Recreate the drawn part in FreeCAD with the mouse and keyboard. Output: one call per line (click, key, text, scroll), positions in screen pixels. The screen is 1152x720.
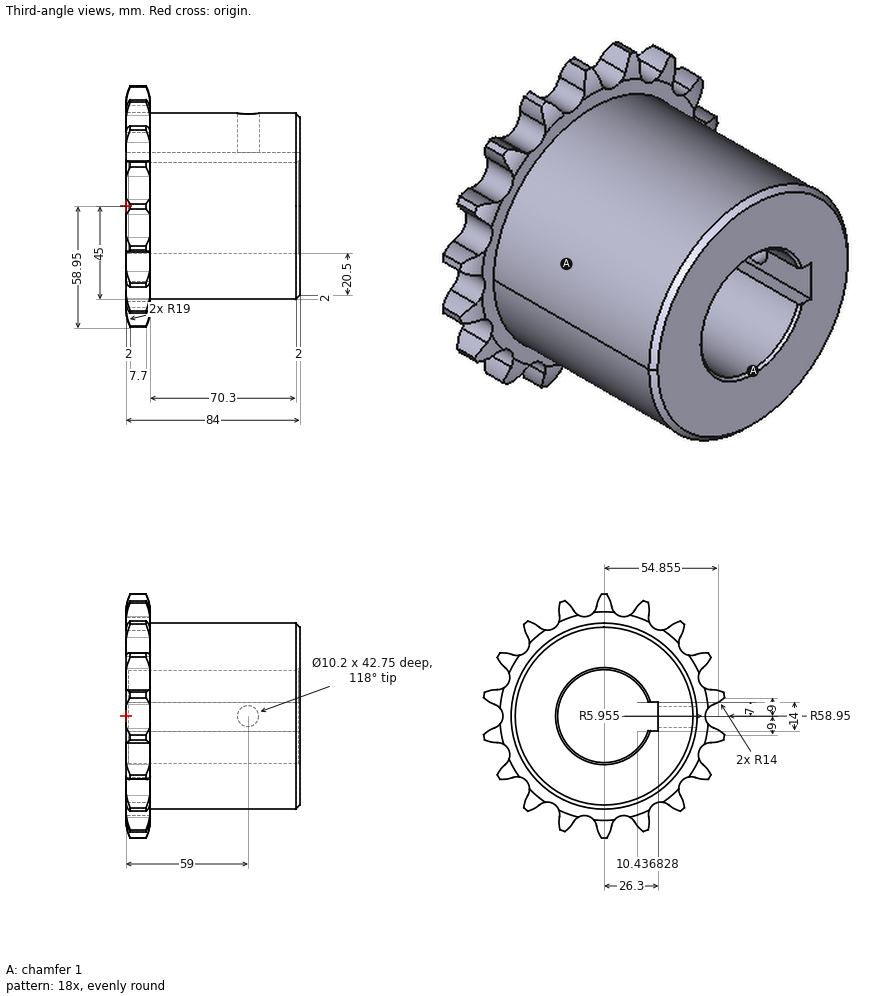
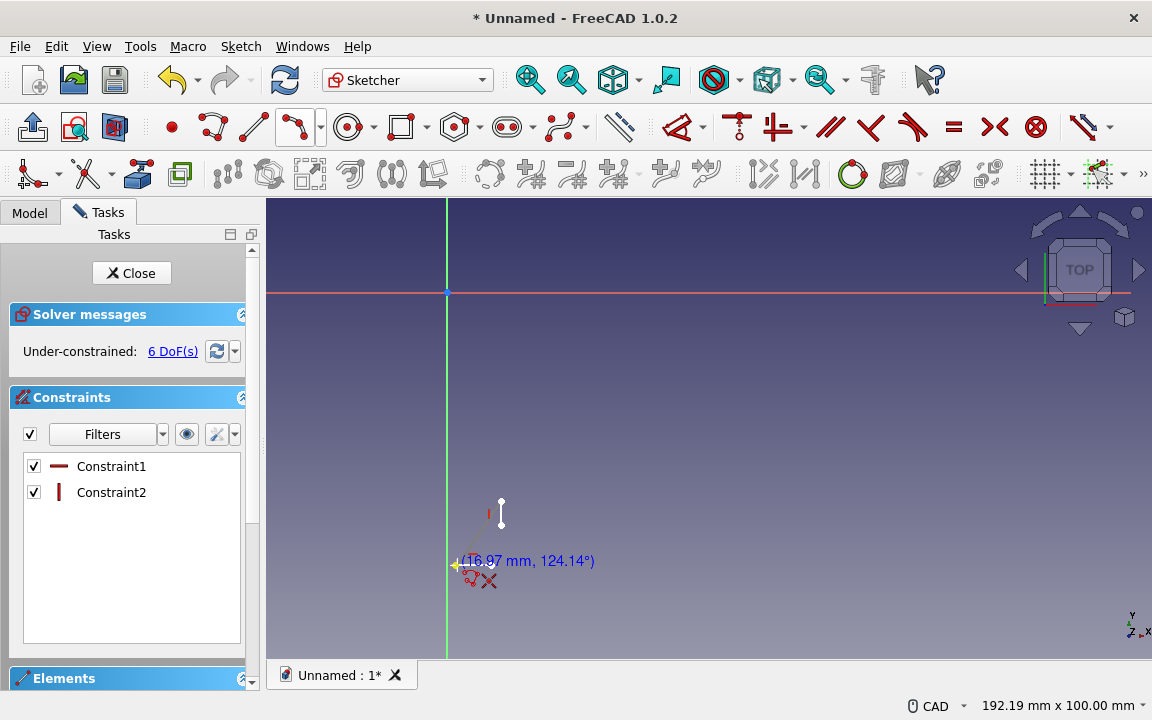
click(825, 501)
click(834, 491)
click(834, 397)
click(447, 397)
click(456, 526)
right_click(456, 526)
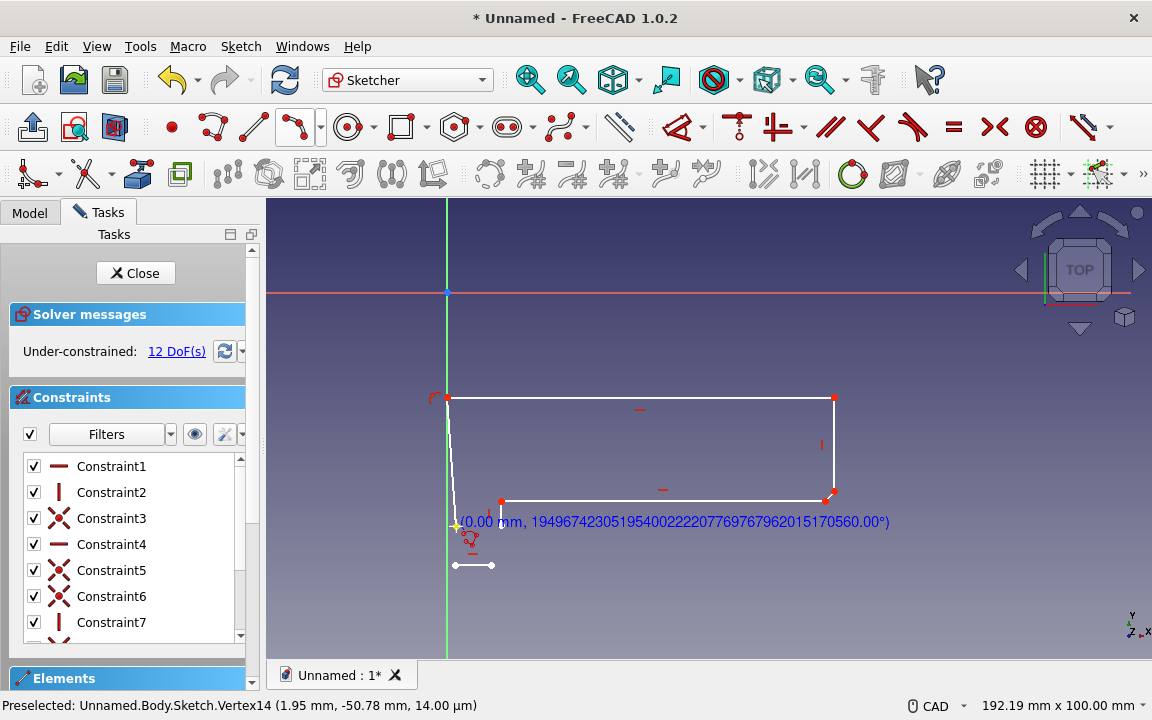
key(g)
key(3)
key(a)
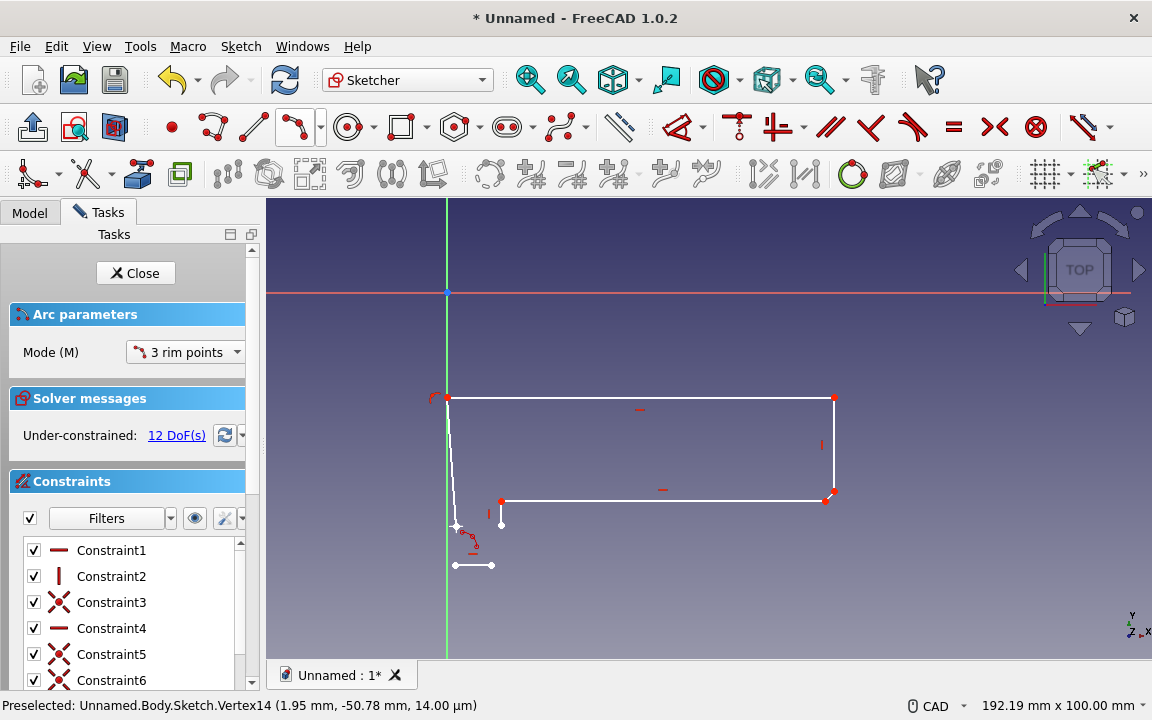
click(492, 565)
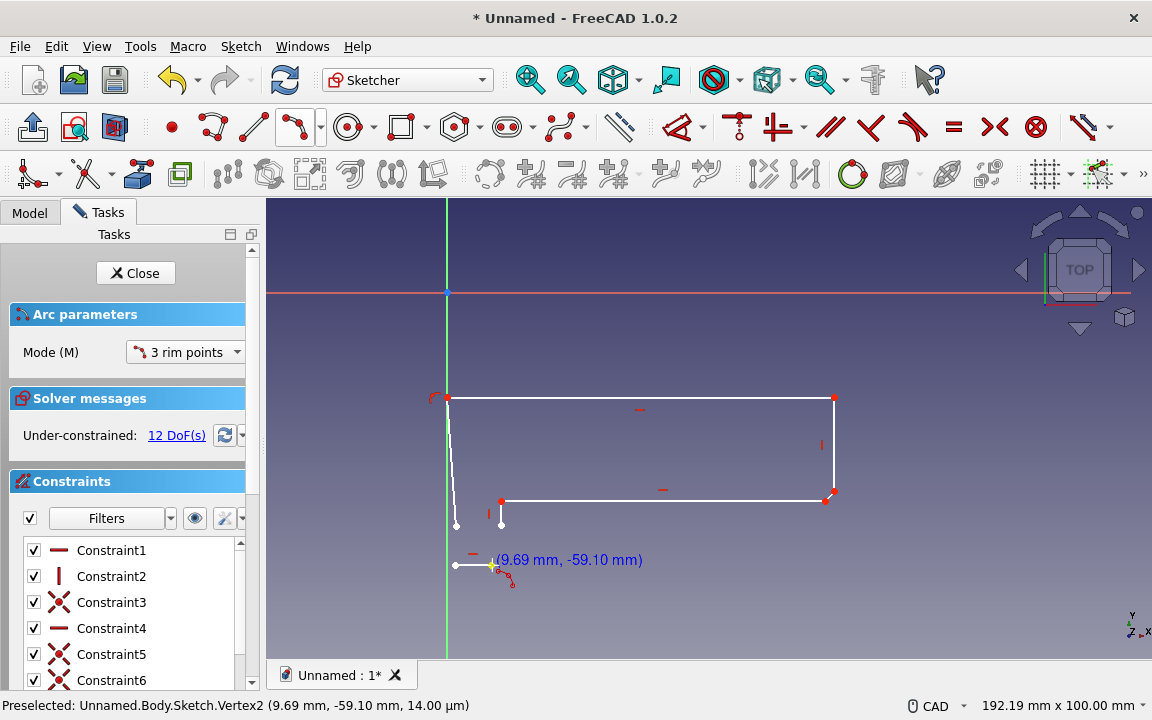
scroll(501, 526, up, 2)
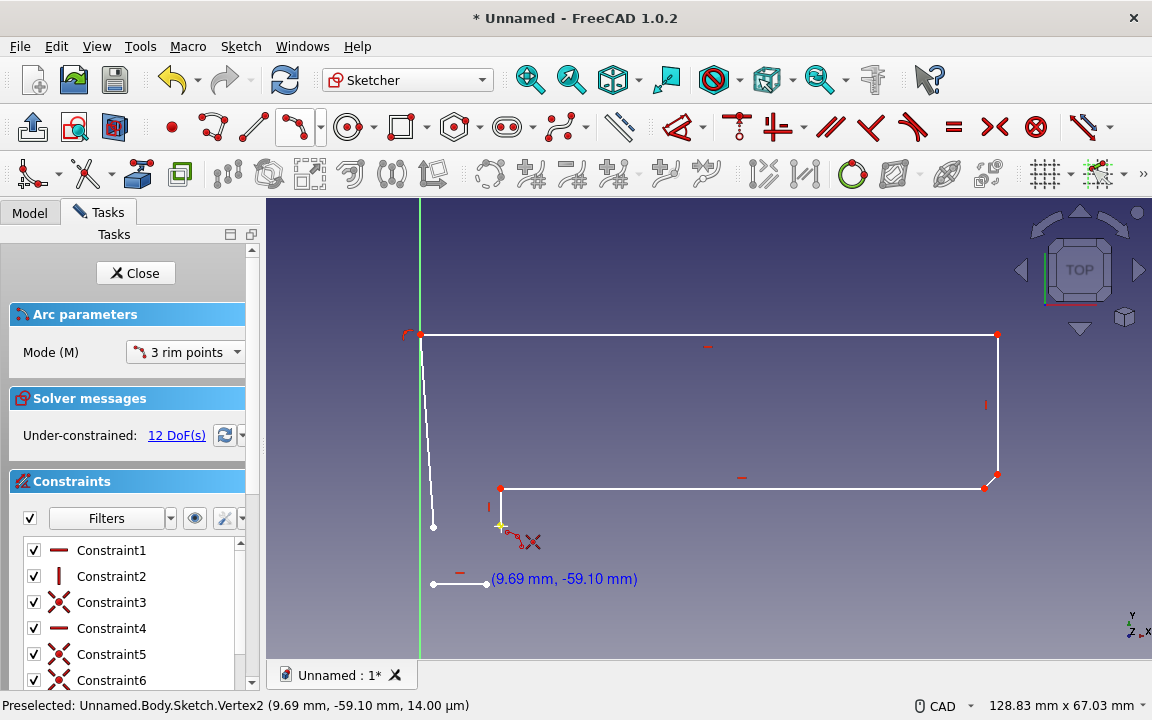
click(501, 525)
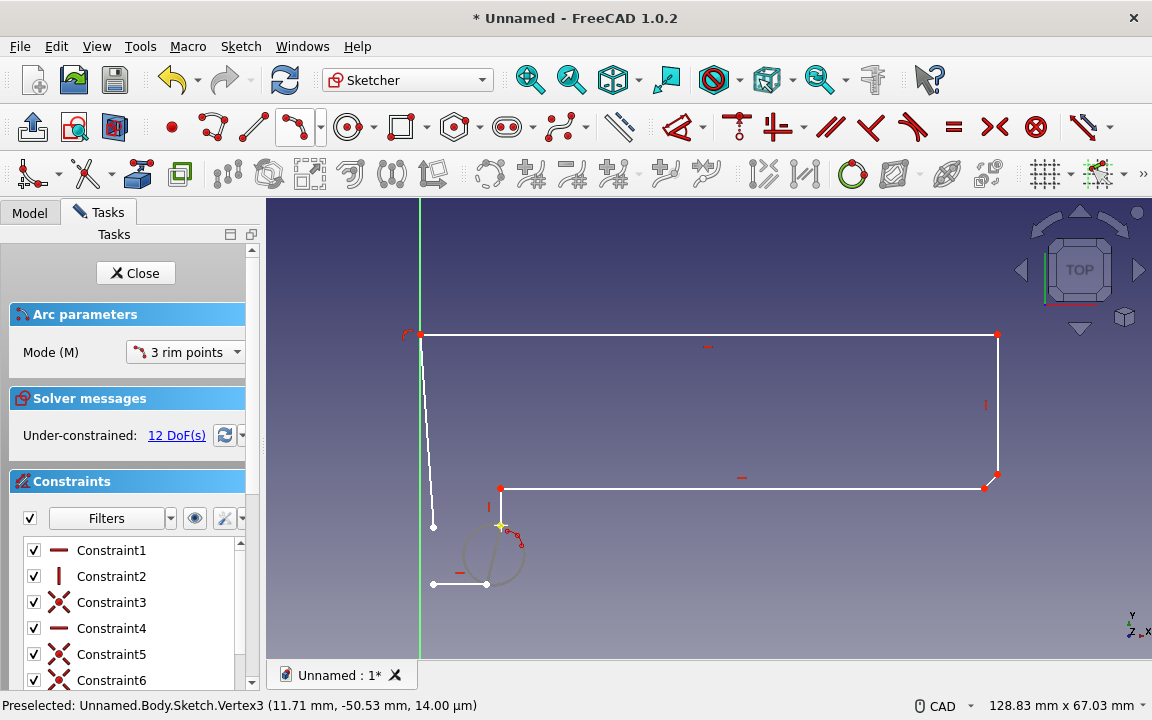
scroll(497, 555, up, 8)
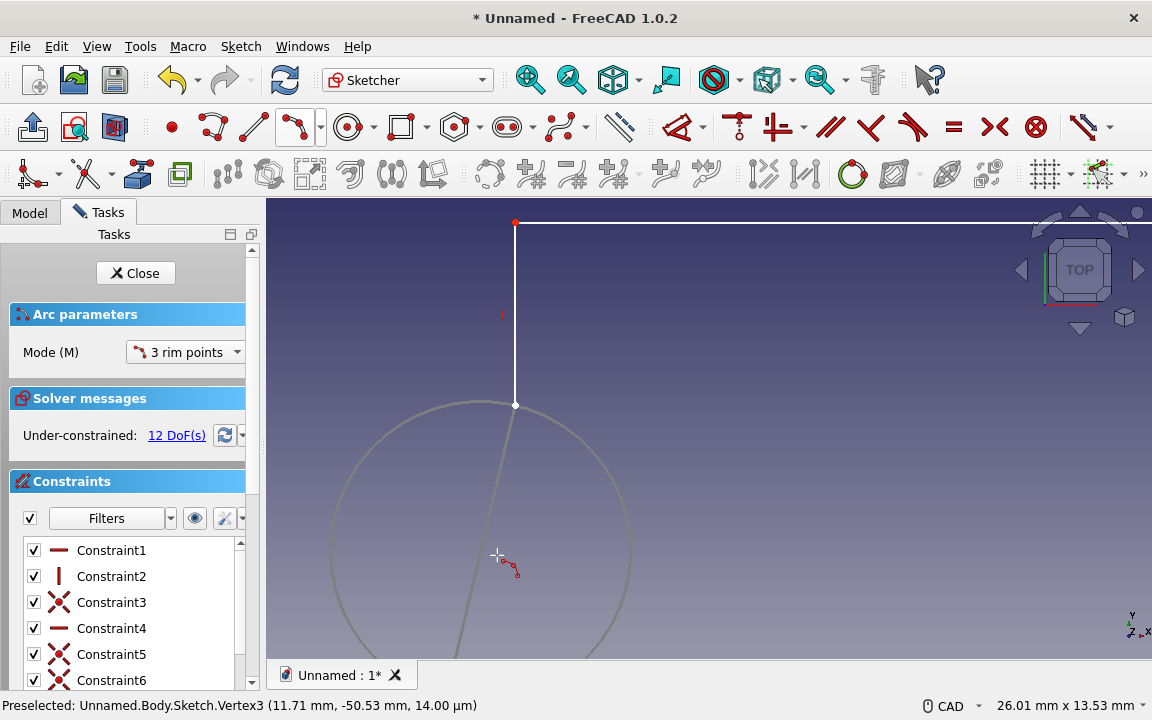
click(498, 552)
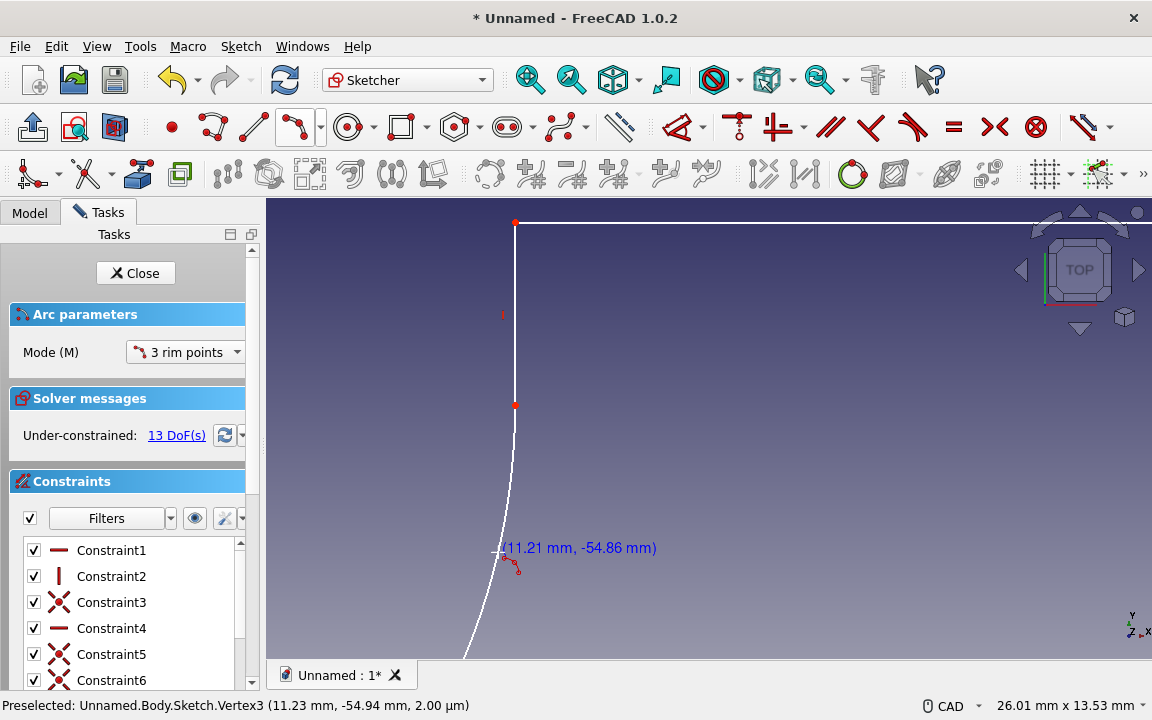
scroll(499, 544, down, 10)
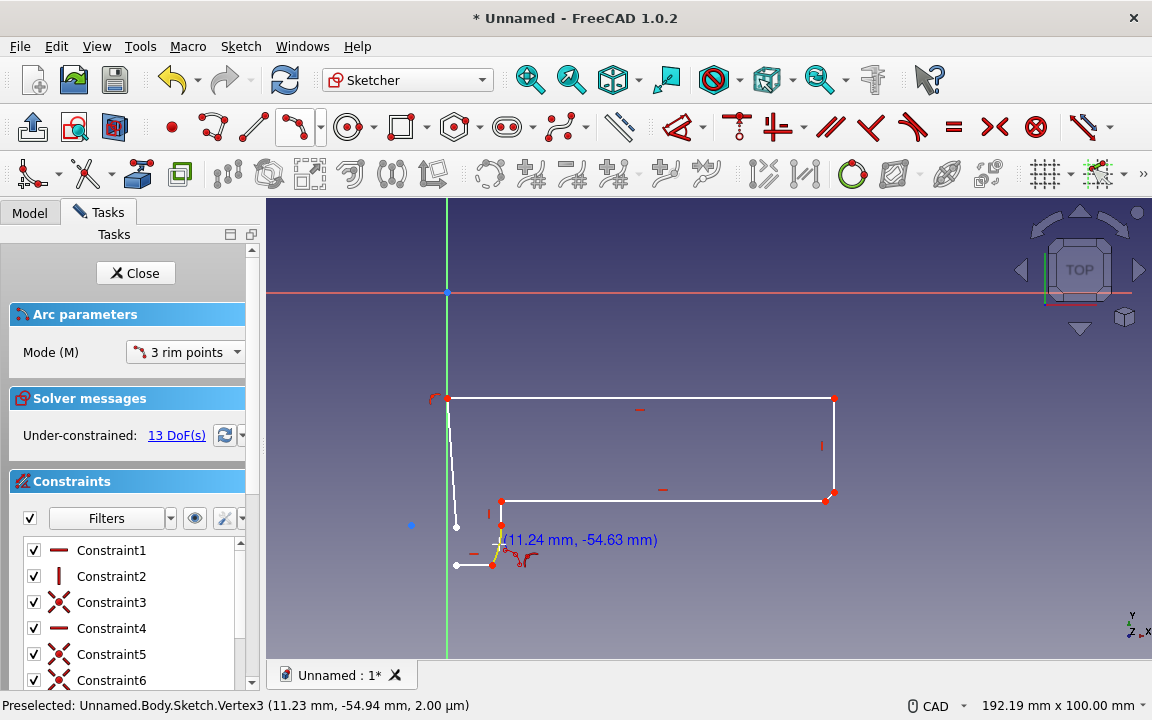
click(456, 527)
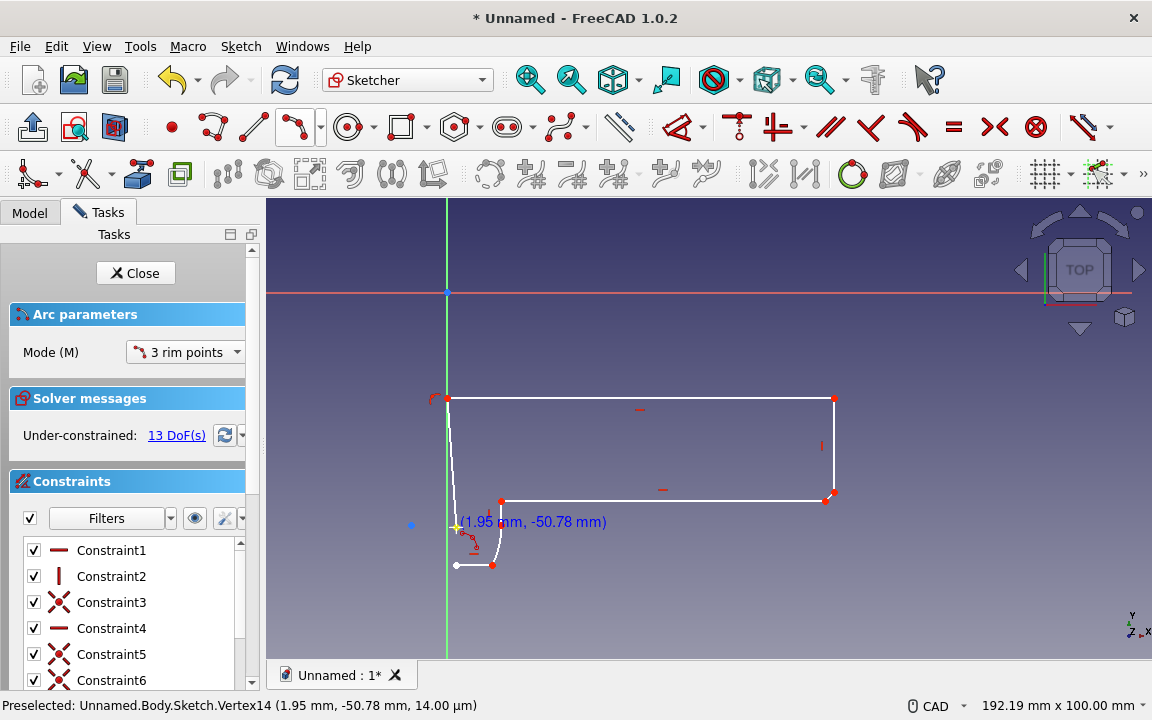
scroll(457, 565, up, 3)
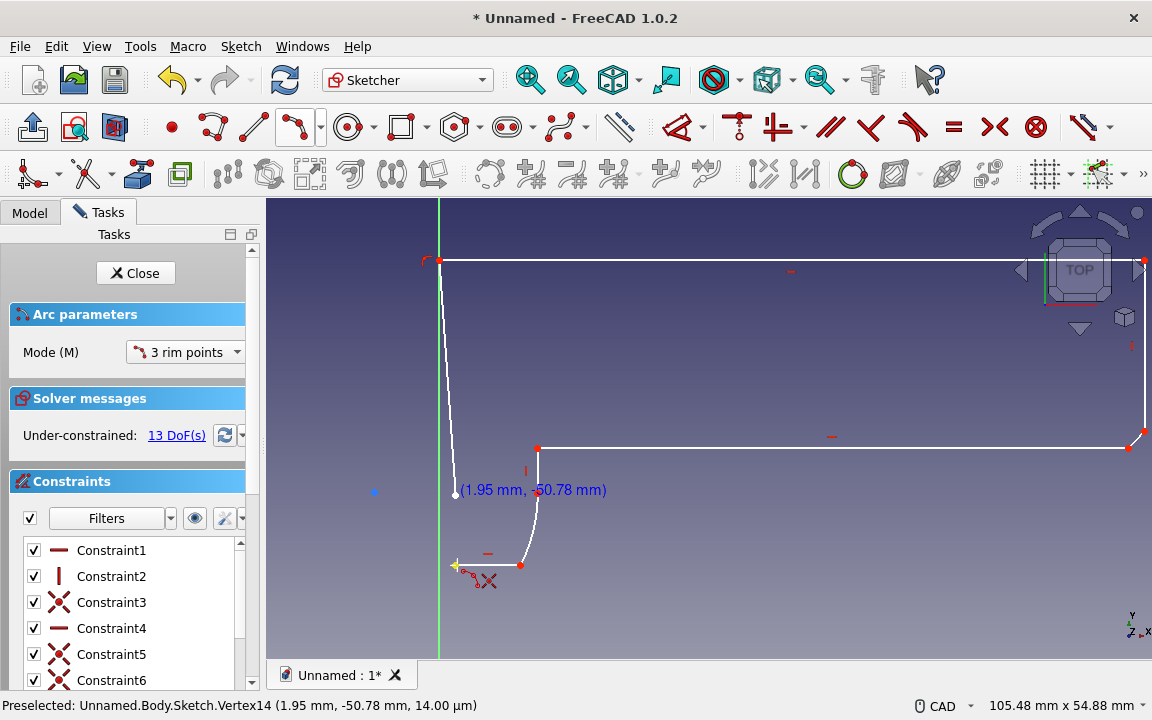
click(456, 565)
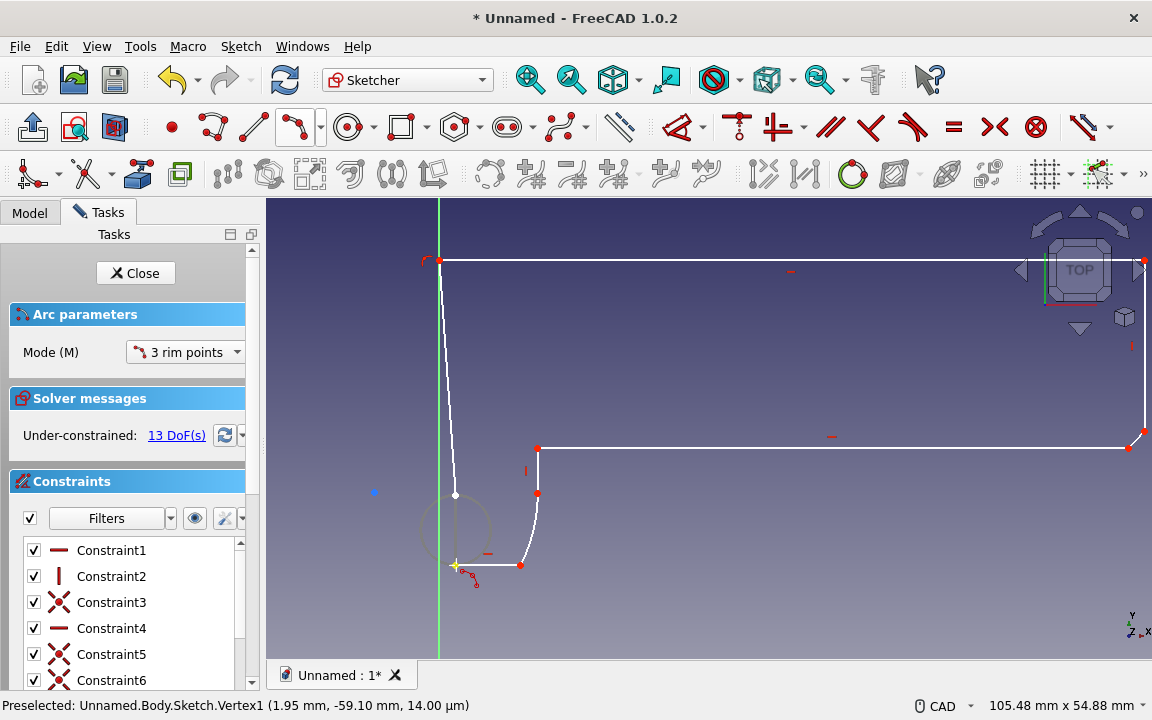
scroll(444, 529, up, 7)